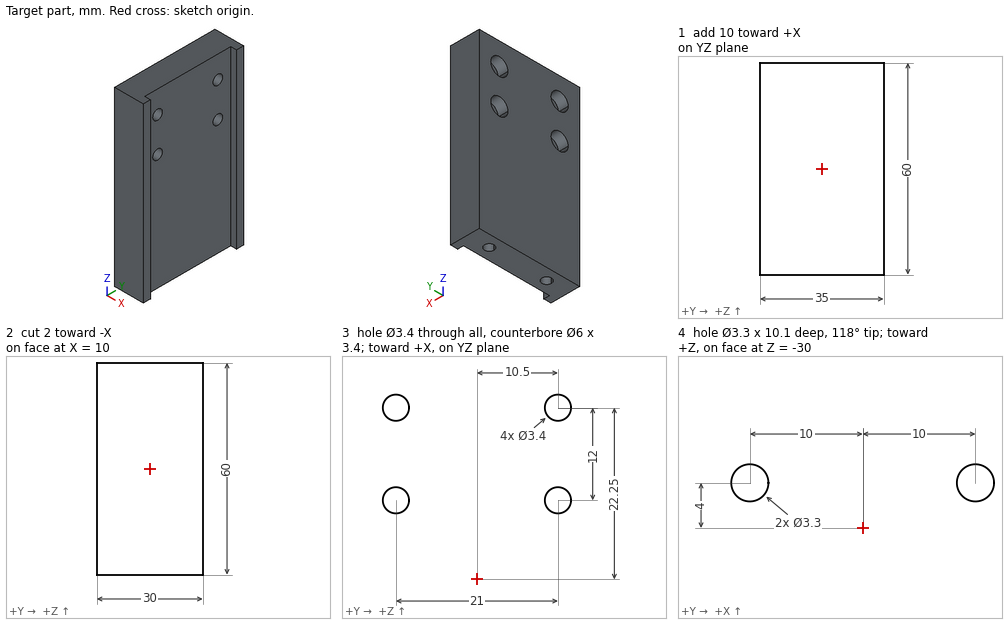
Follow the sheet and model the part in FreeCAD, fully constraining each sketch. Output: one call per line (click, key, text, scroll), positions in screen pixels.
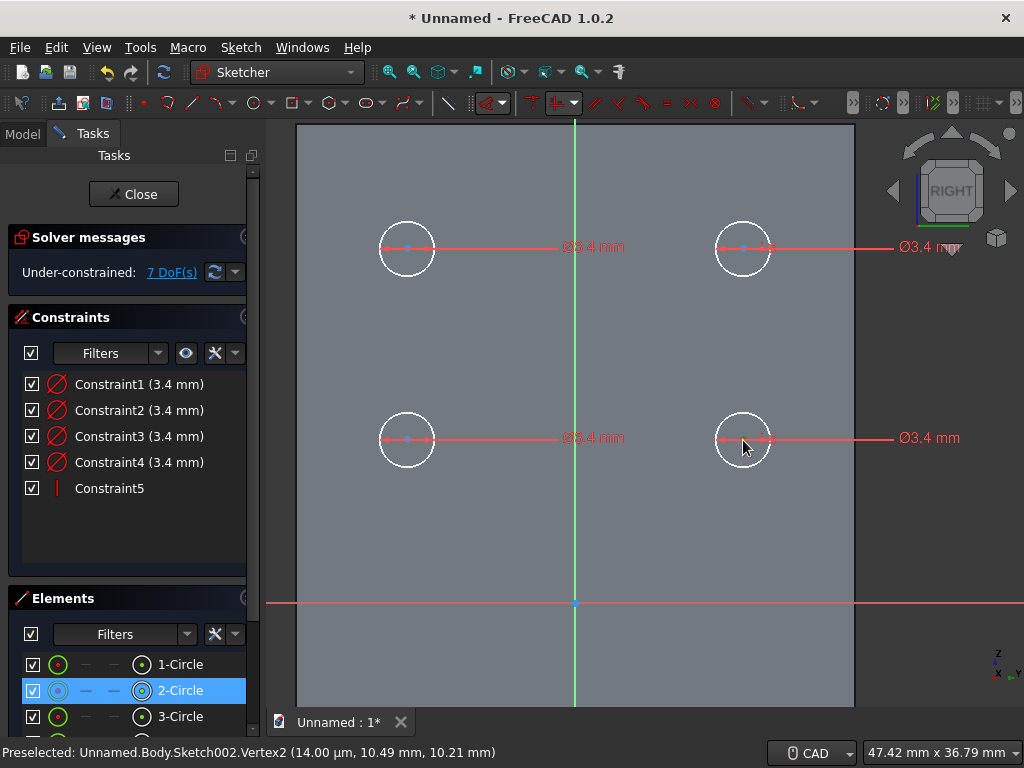
click(407, 440)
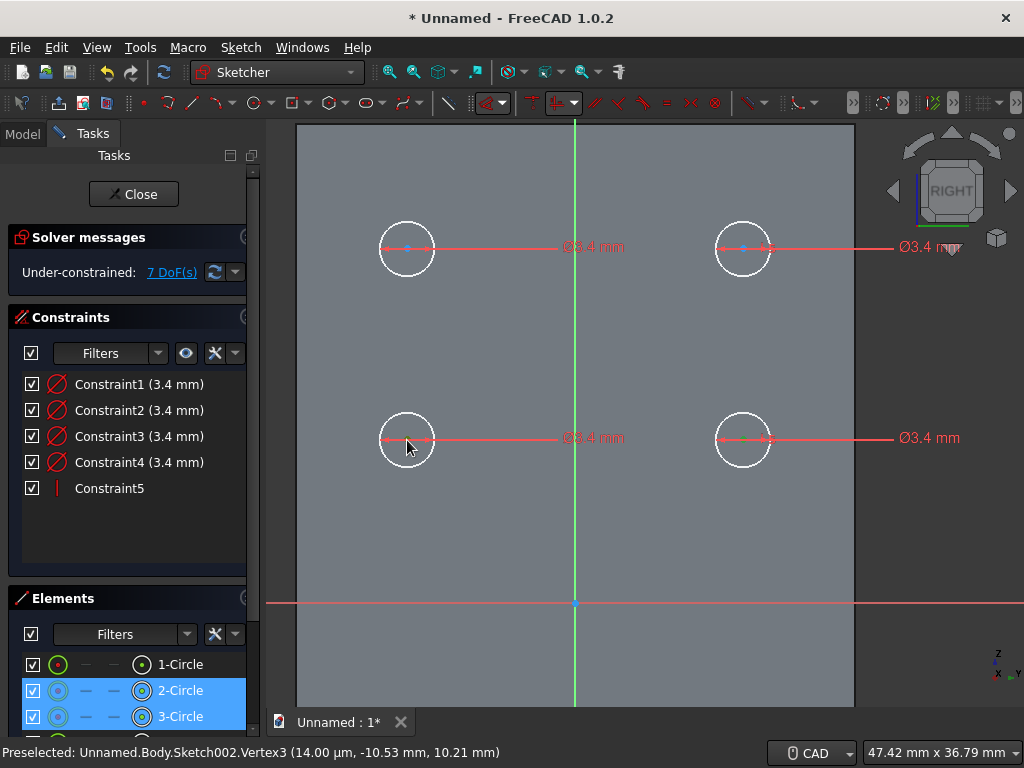
key(h)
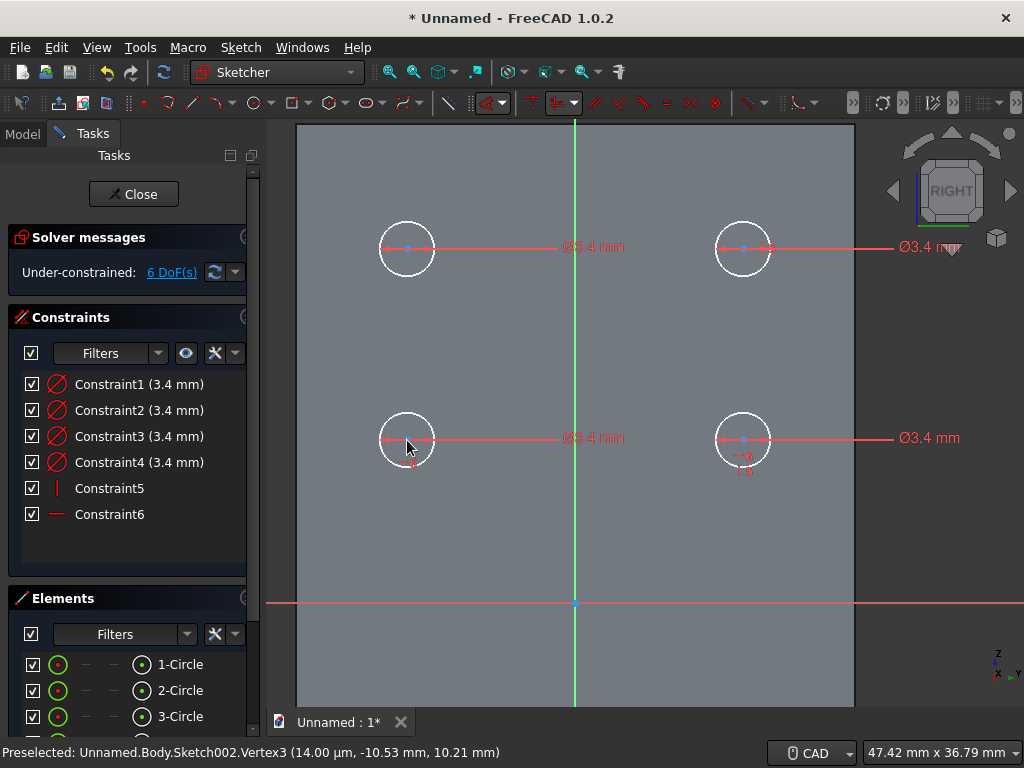
click(407, 440)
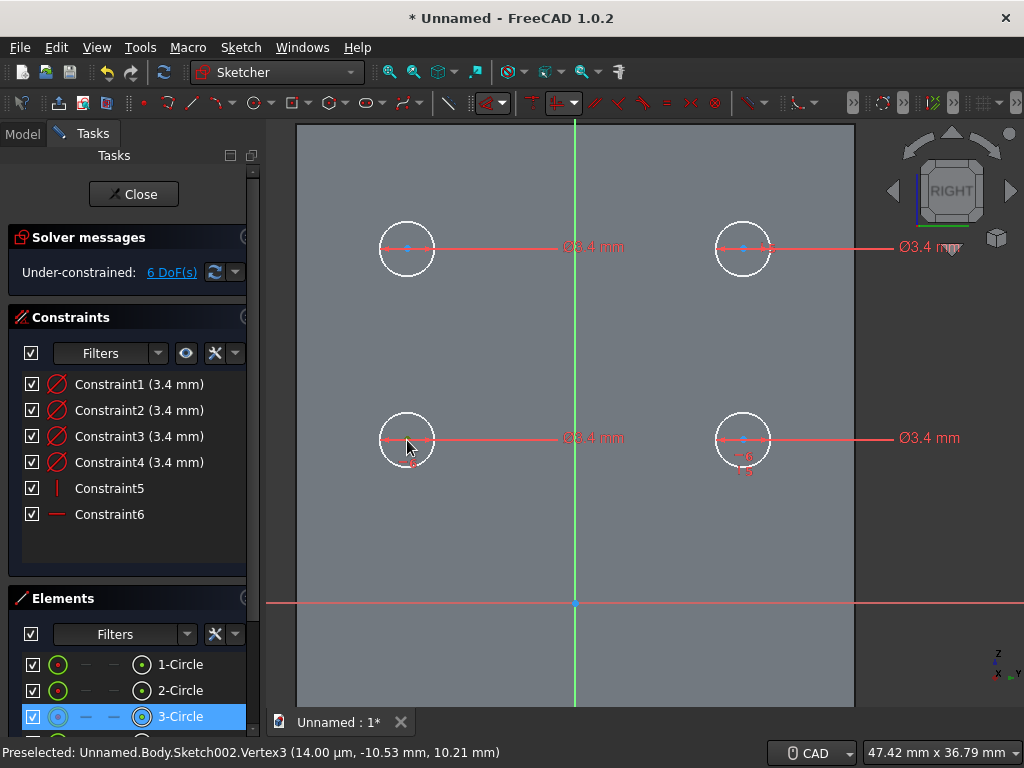
click(407, 249)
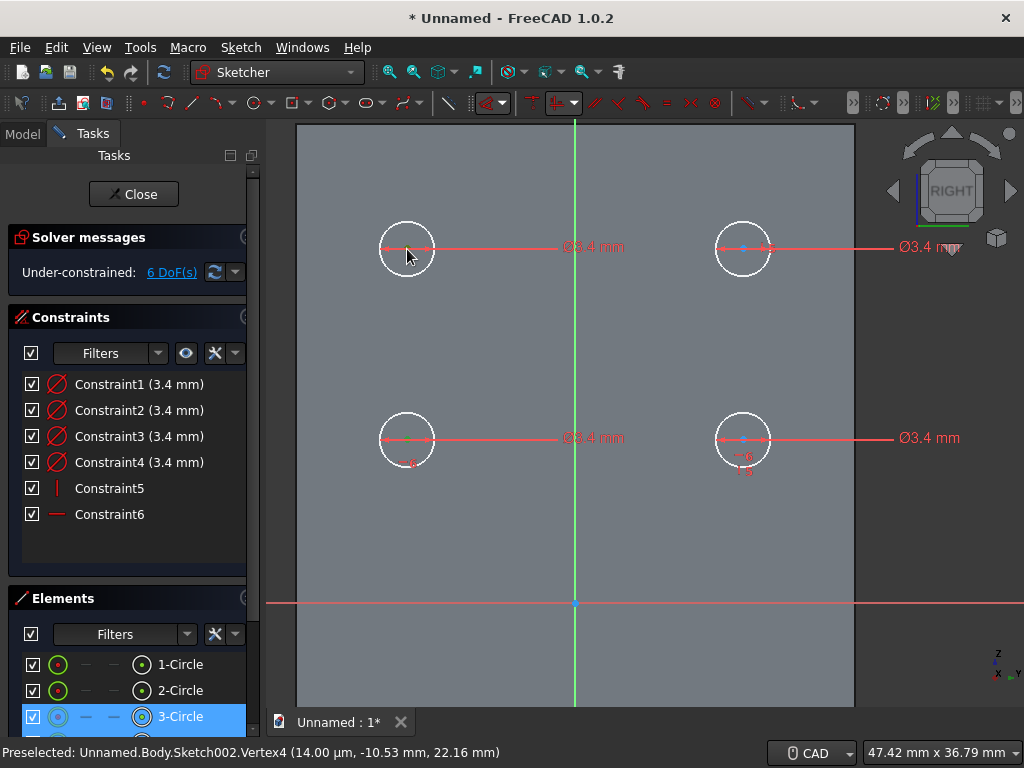
click(576, 104)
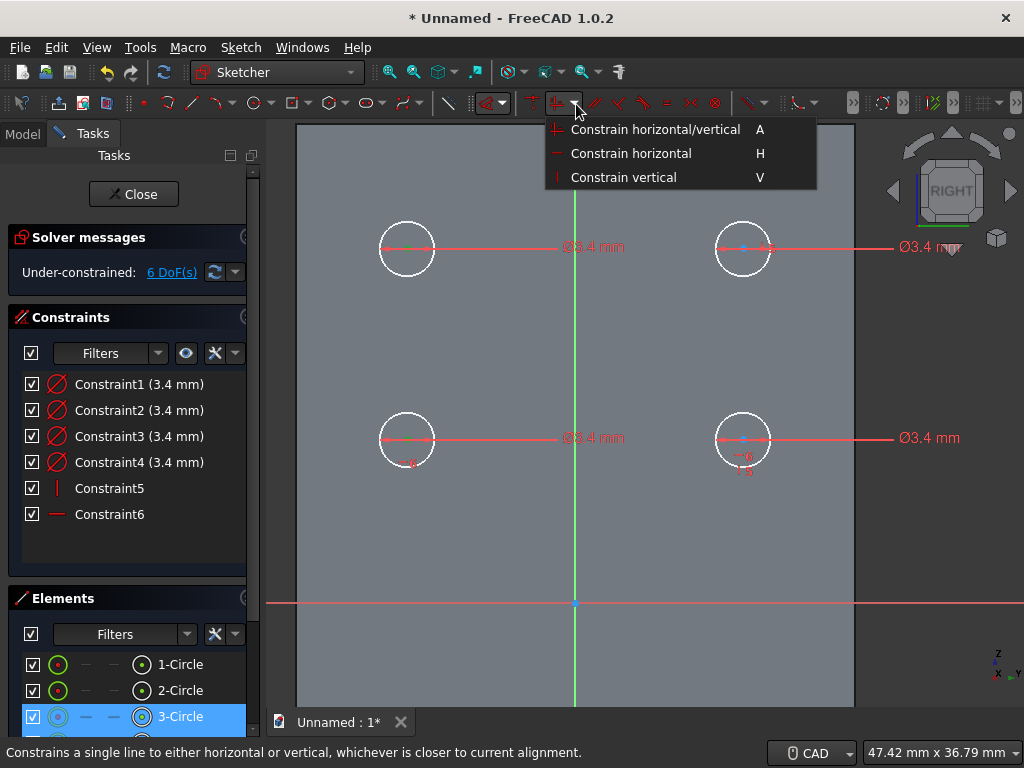
click(681, 177)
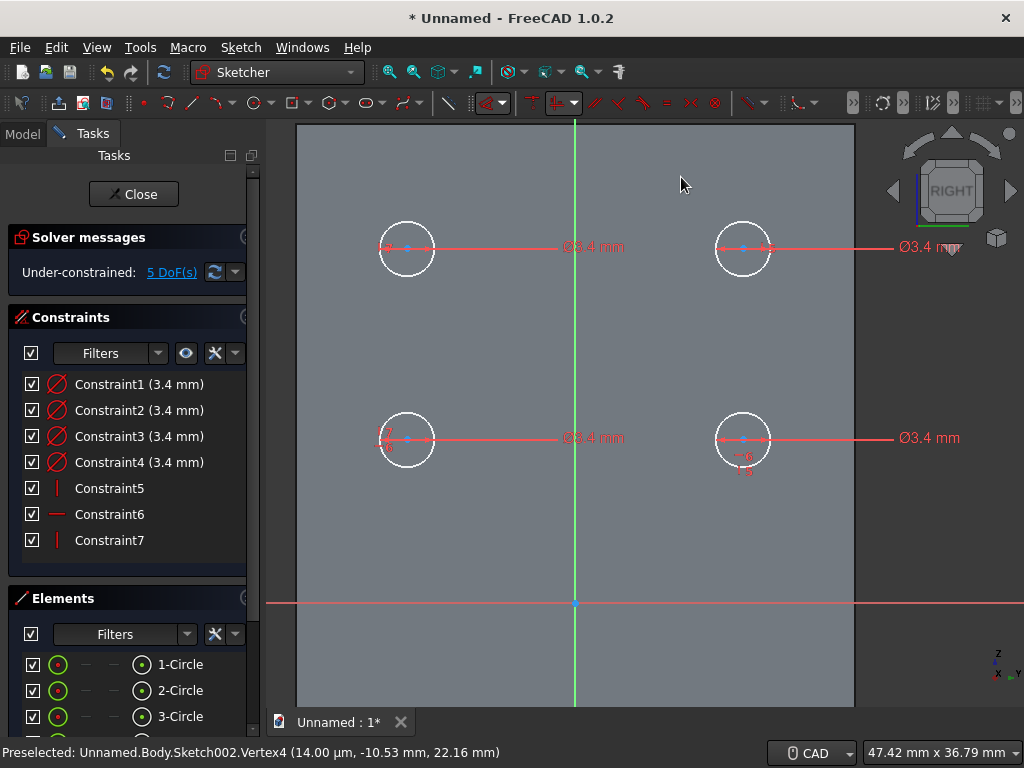
click(743, 249)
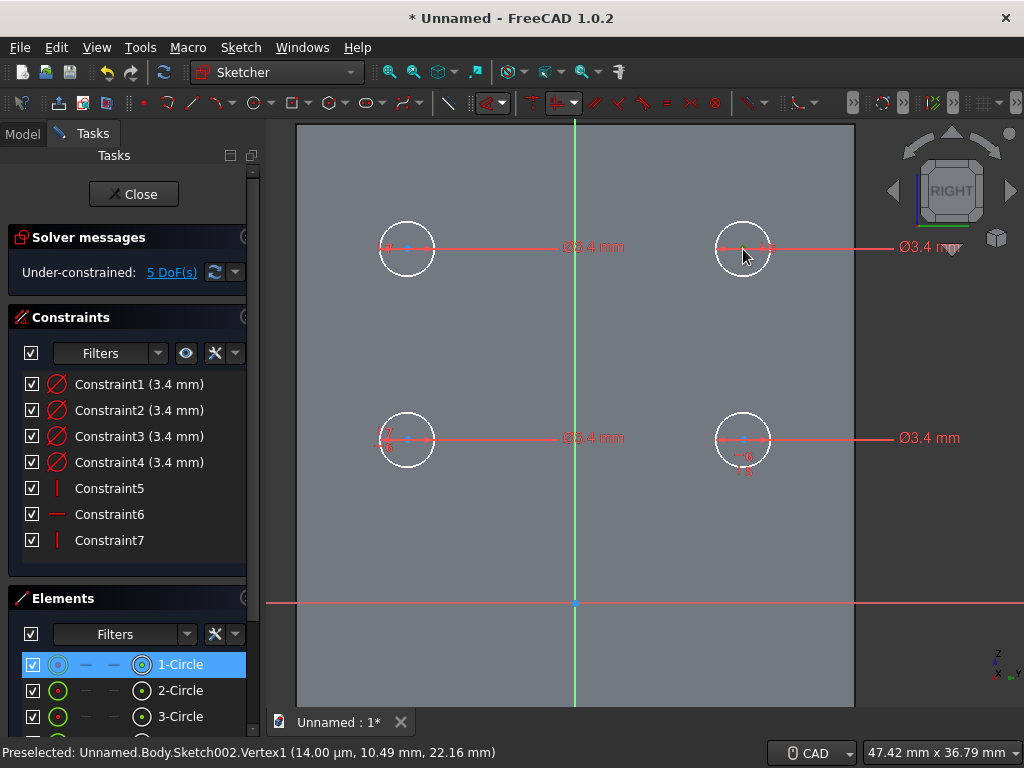
click(407, 249)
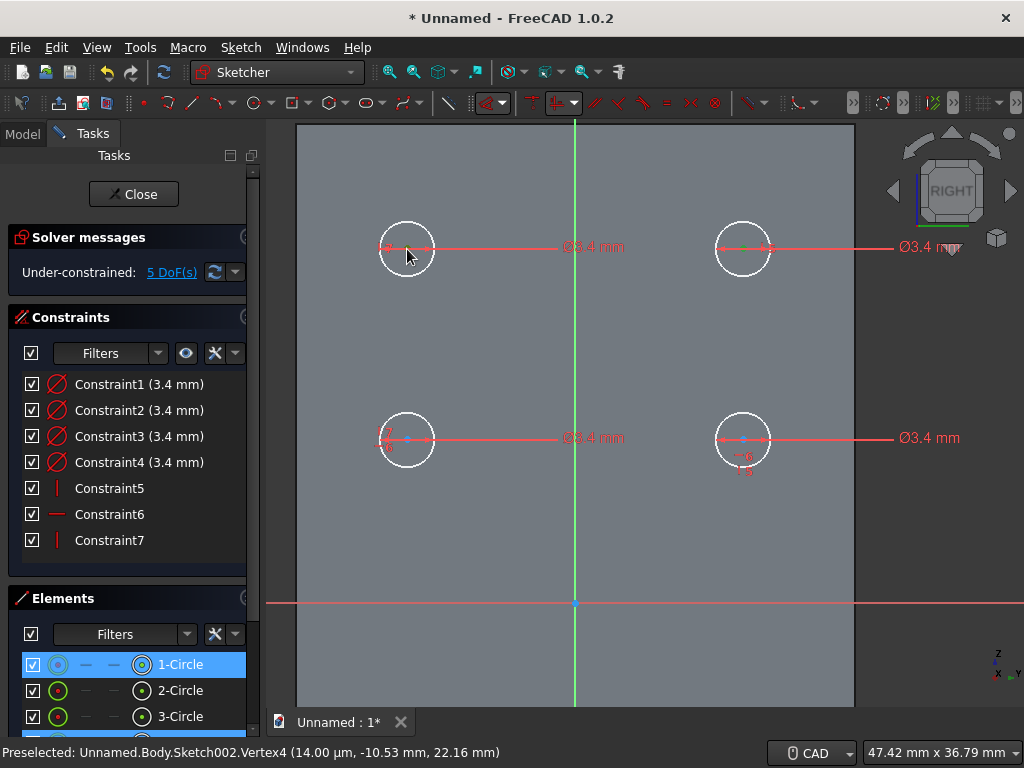
key(h)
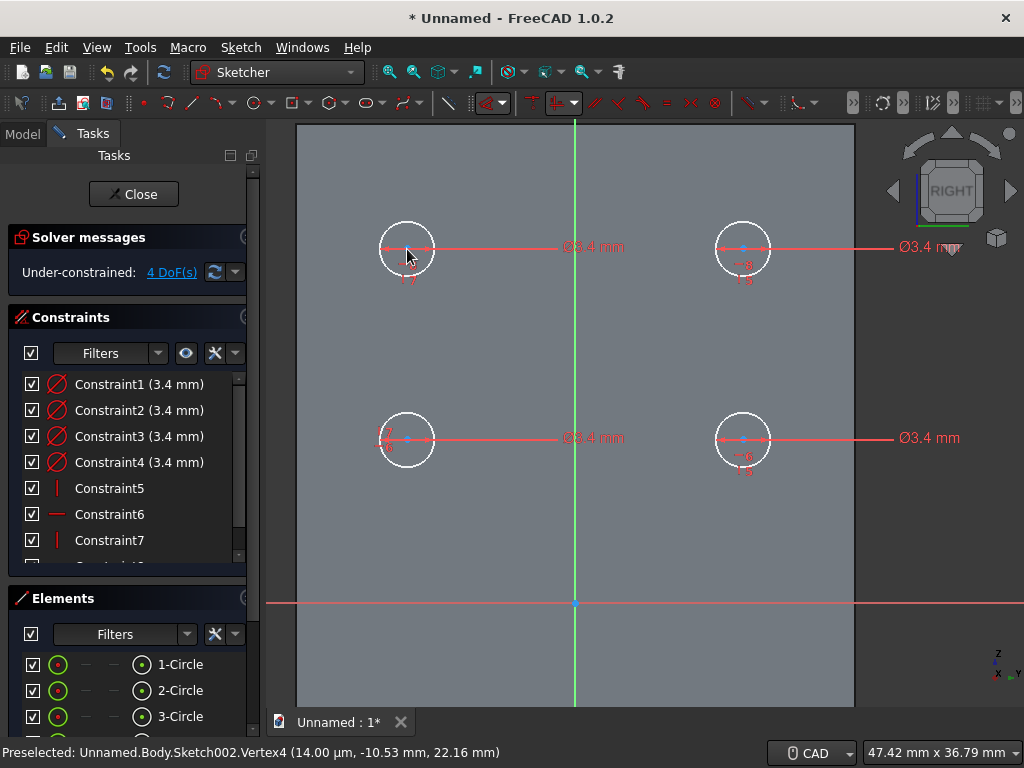
click(486, 104)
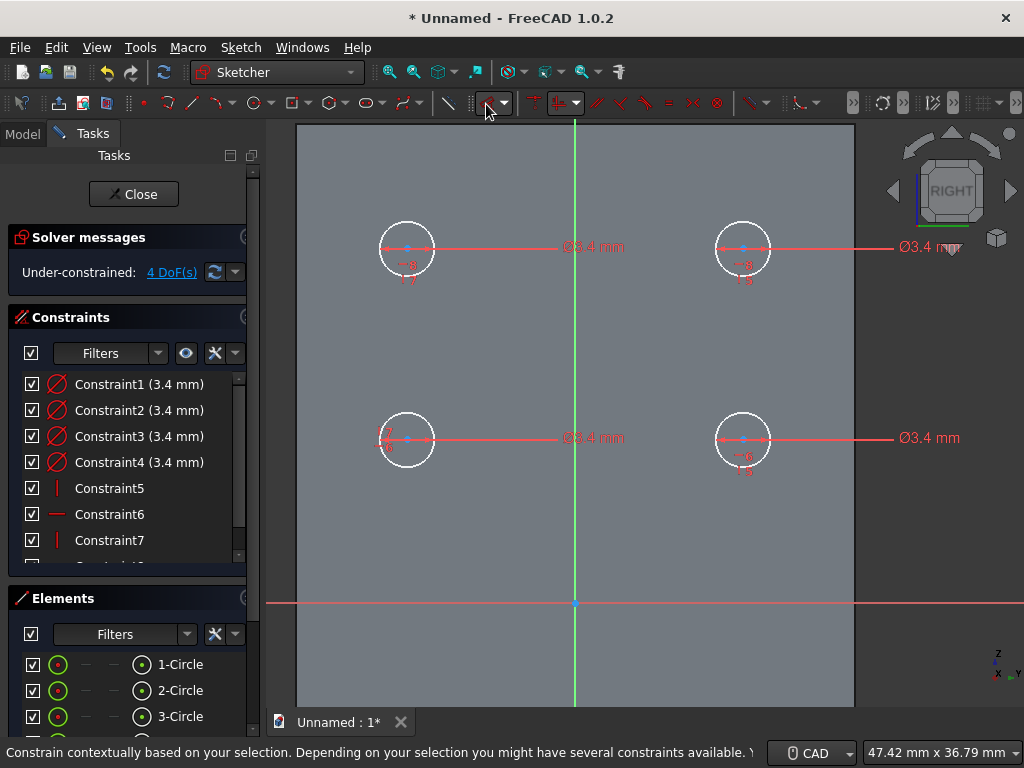
click(743, 249)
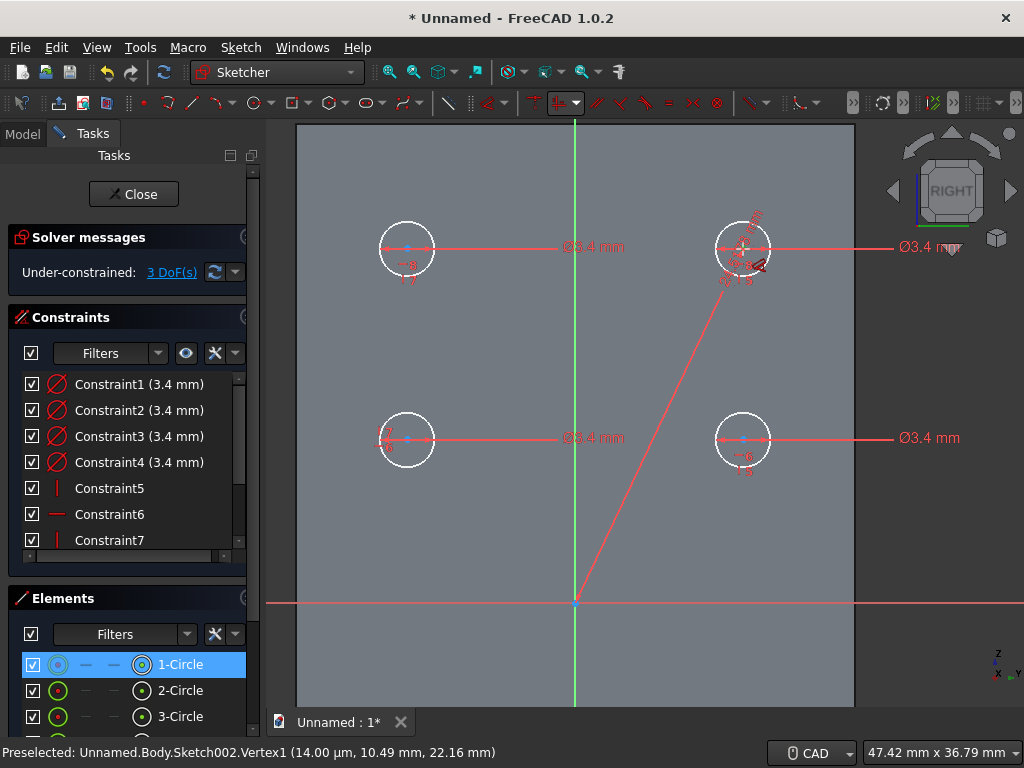
click(743, 440)
click(777, 344)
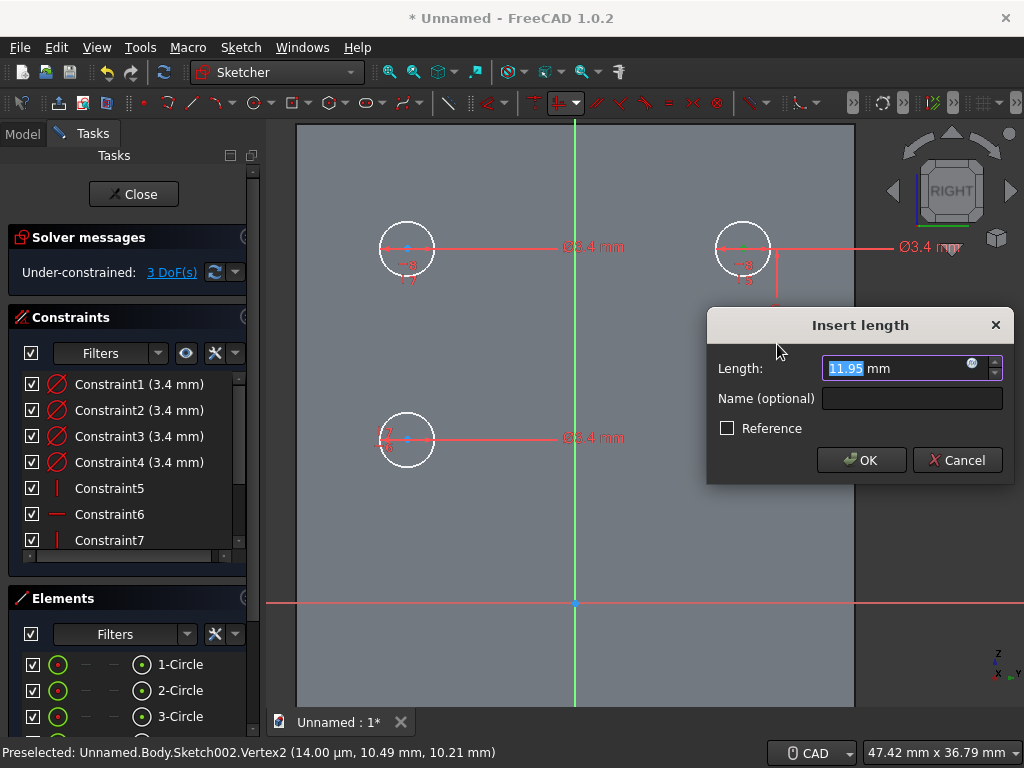
text(12)
key(Return)